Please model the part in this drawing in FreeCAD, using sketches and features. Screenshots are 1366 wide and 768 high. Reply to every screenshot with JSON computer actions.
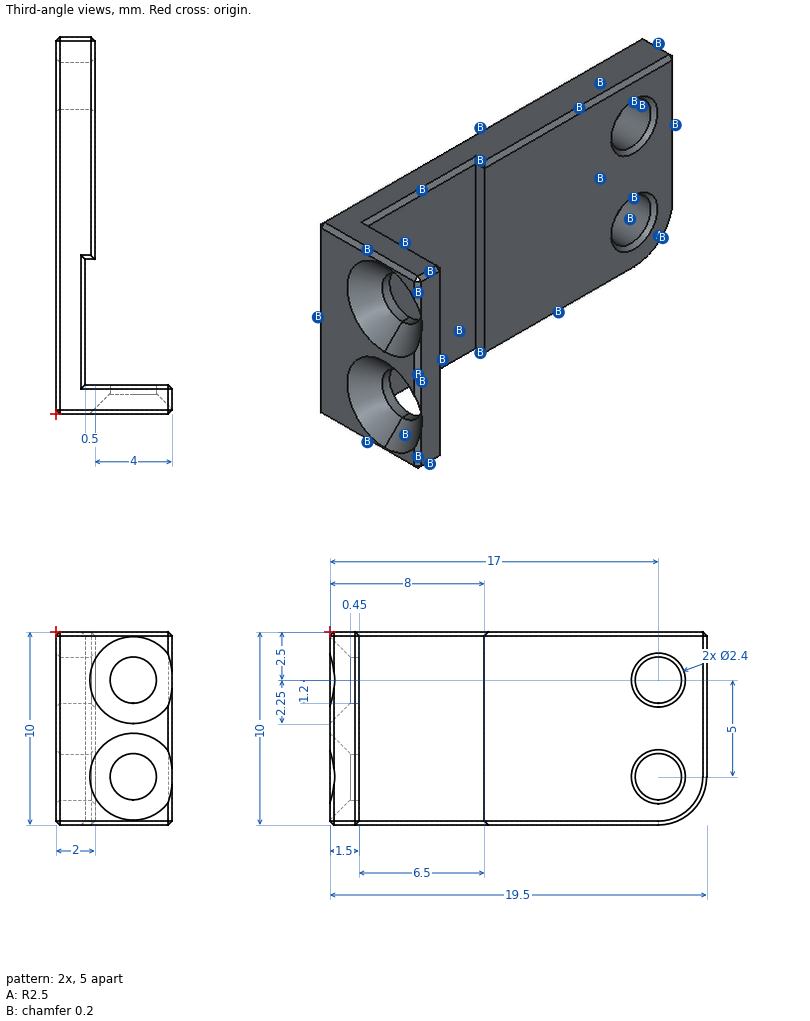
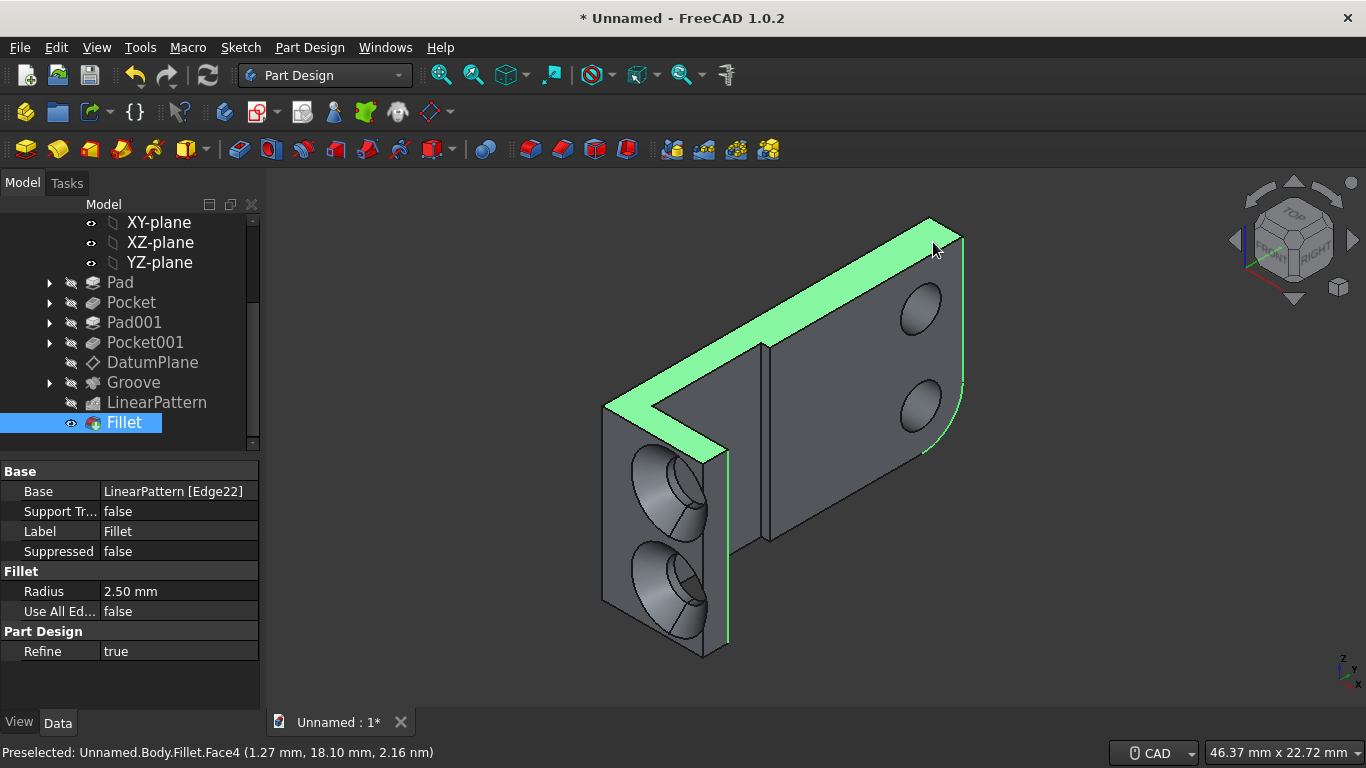
{"action": "left_click", "coordinate": [703, 560], "text": "ctrl"}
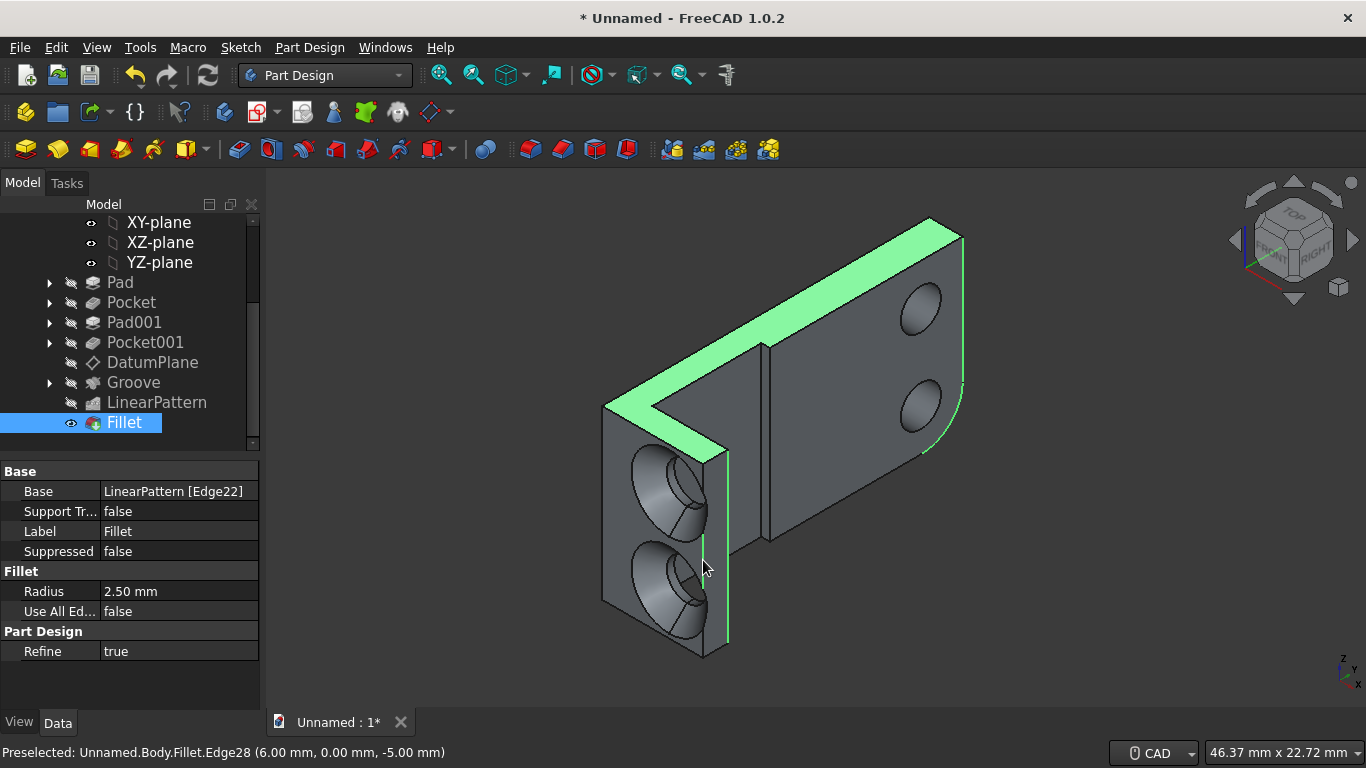
{"action": "left_click", "coordinate": [703, 643], "text": "ctrl"}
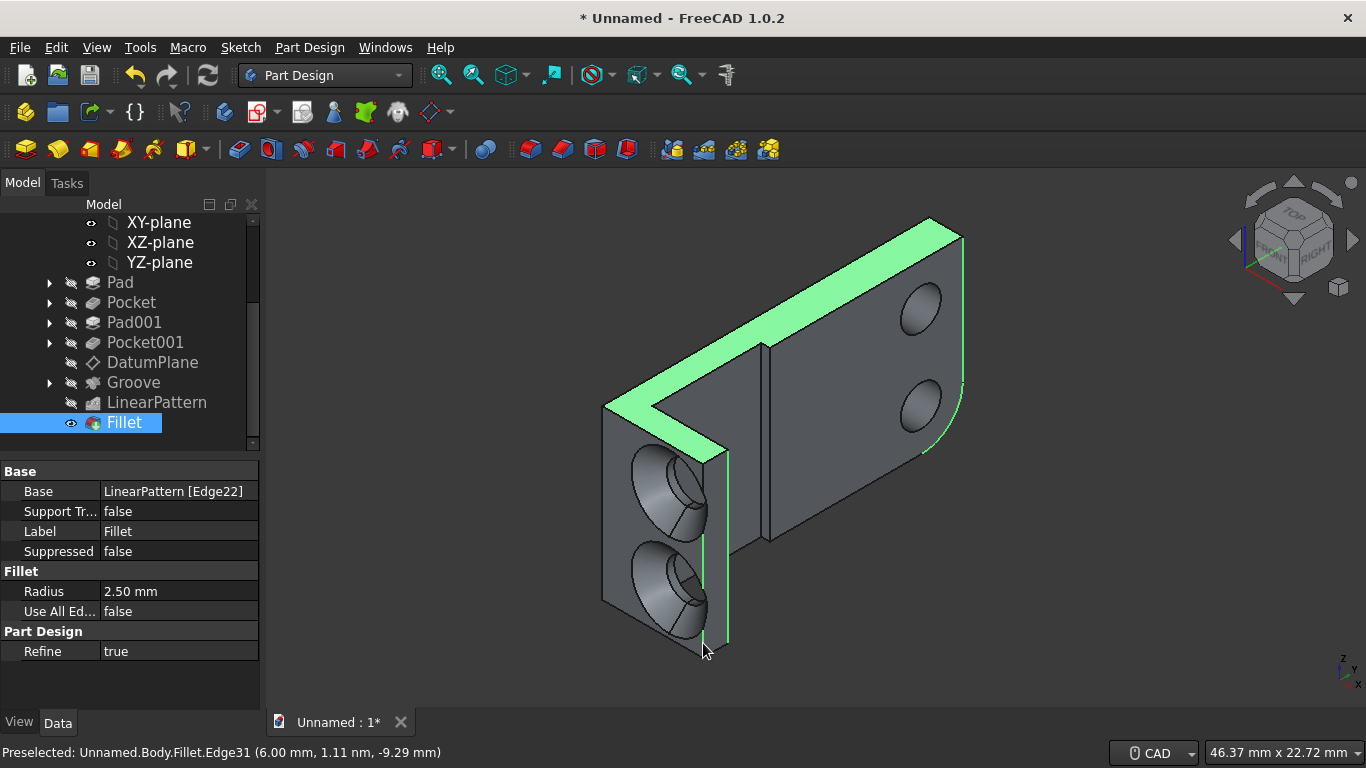
{"action": "left_click", "coordinate": [703, 477], "text": "ctrl"}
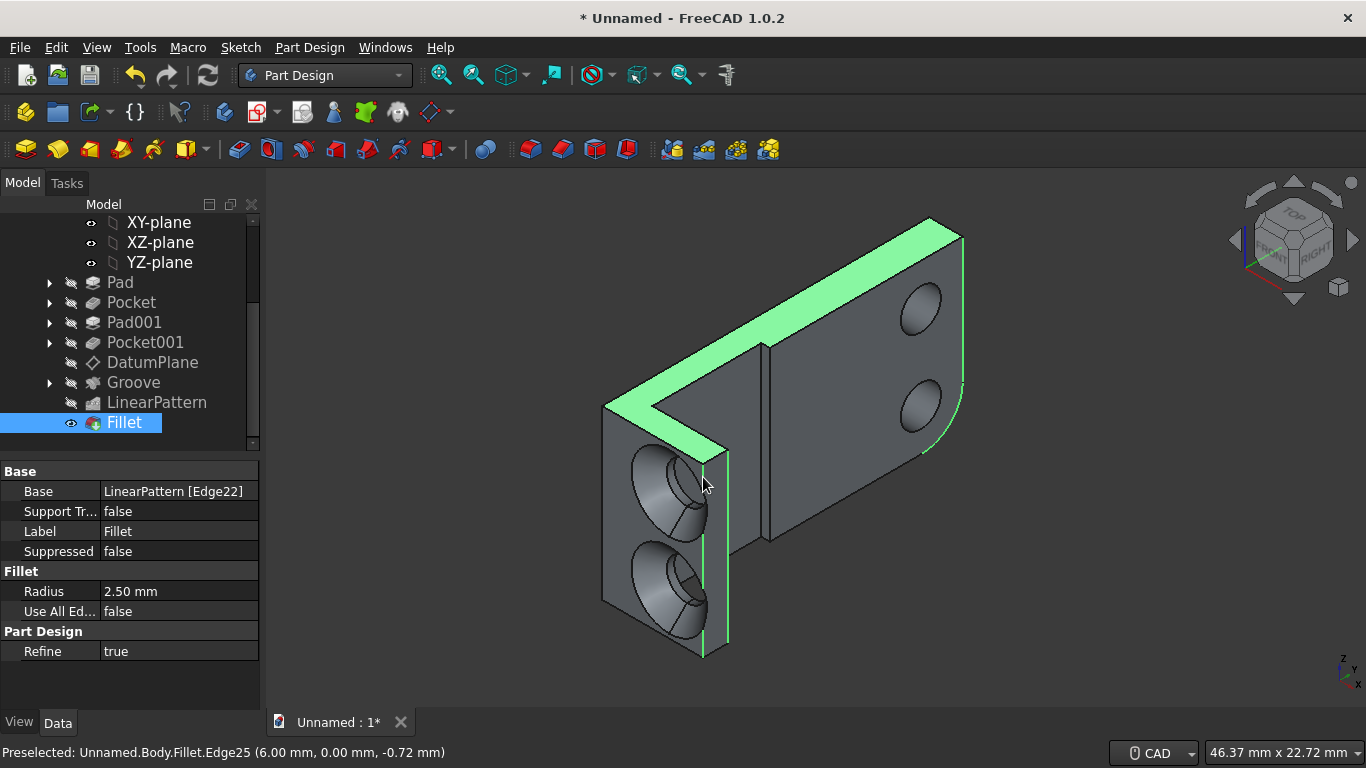
{"action": "left_click", "coordinate": [921, 331], "text": "ctrl"}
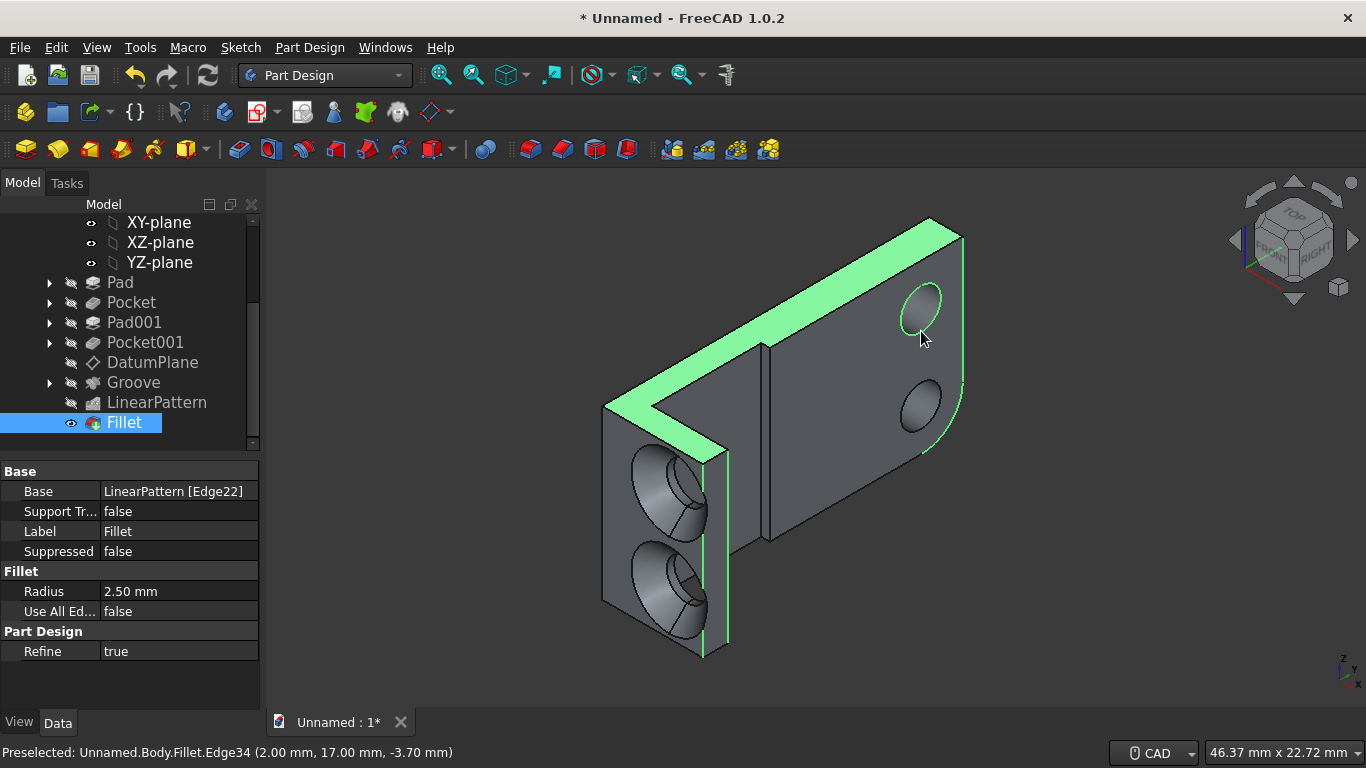
{"action": "left_click", "coordinate": [921, 428], "text": "ctrl"}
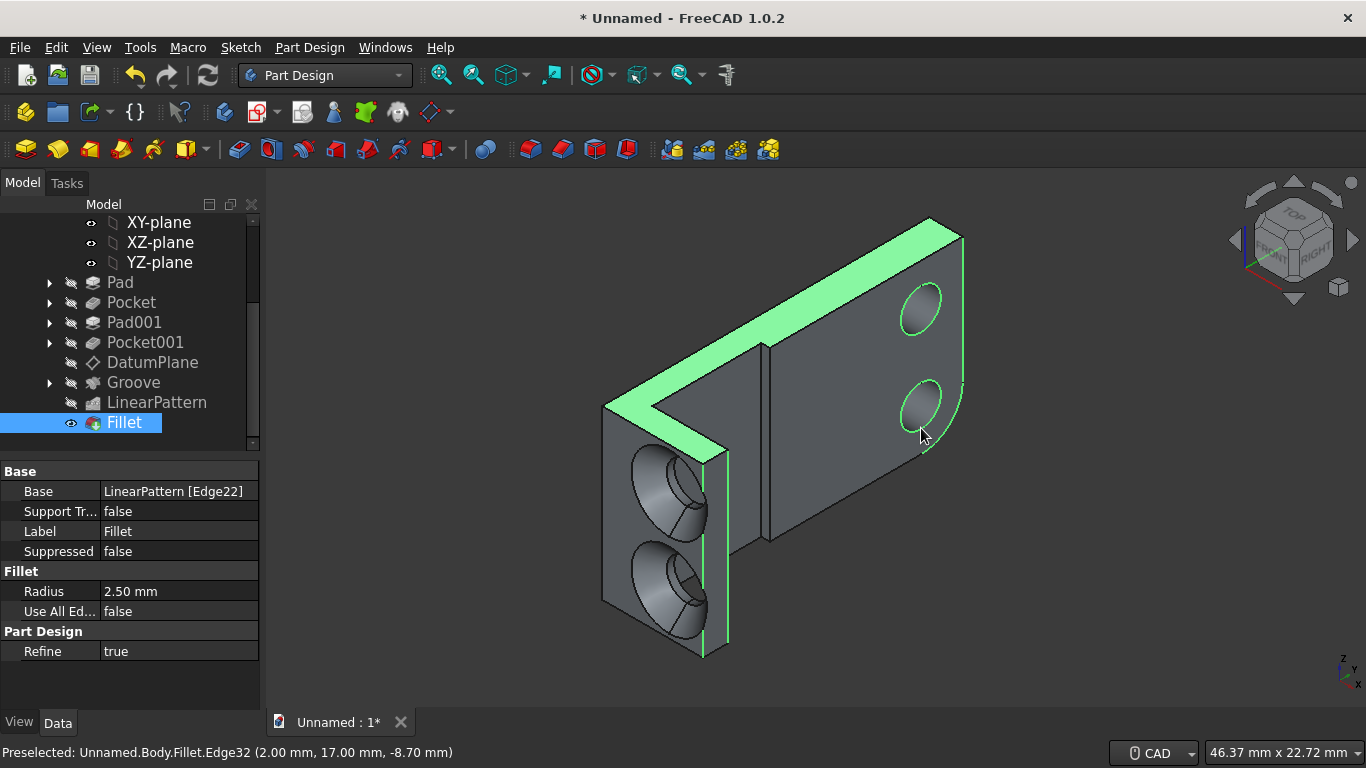
{"action": "key", "text": "2"}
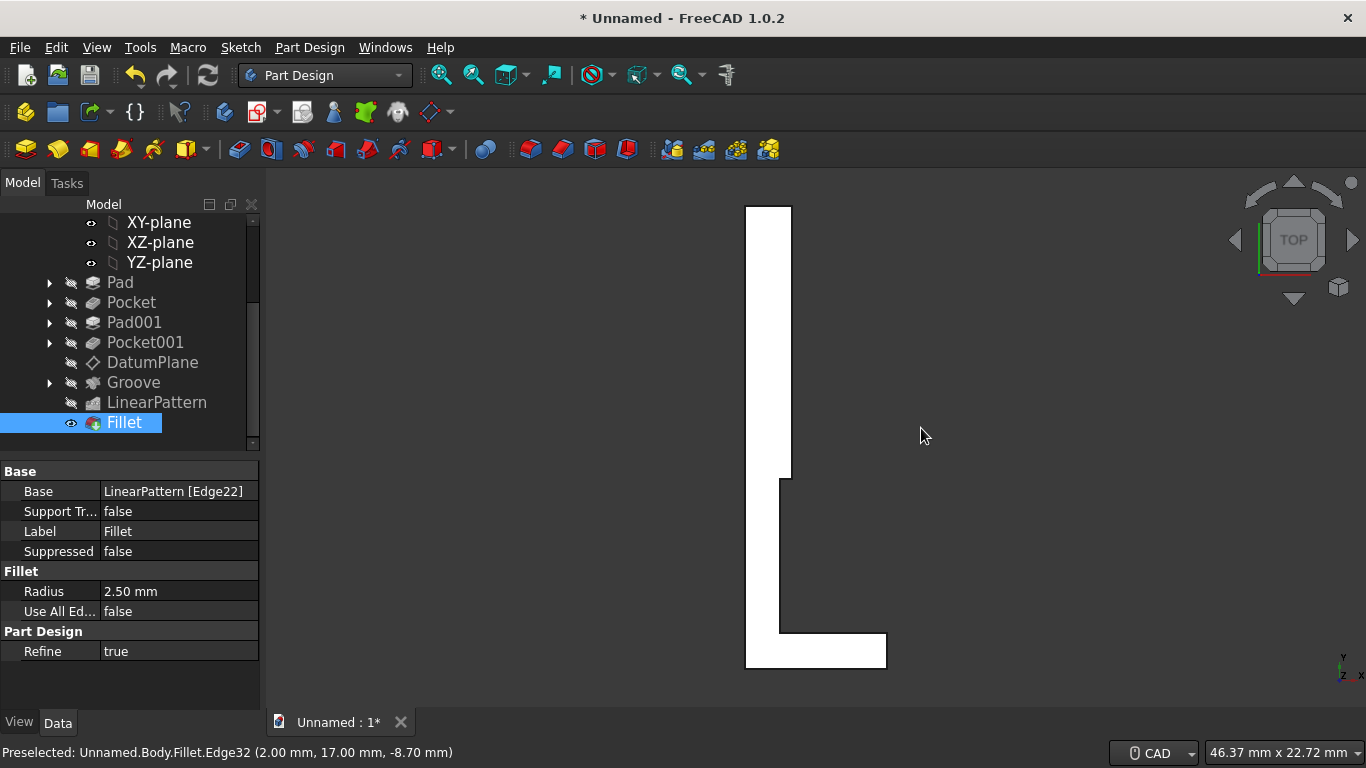
{"action": "key", "text": "1"}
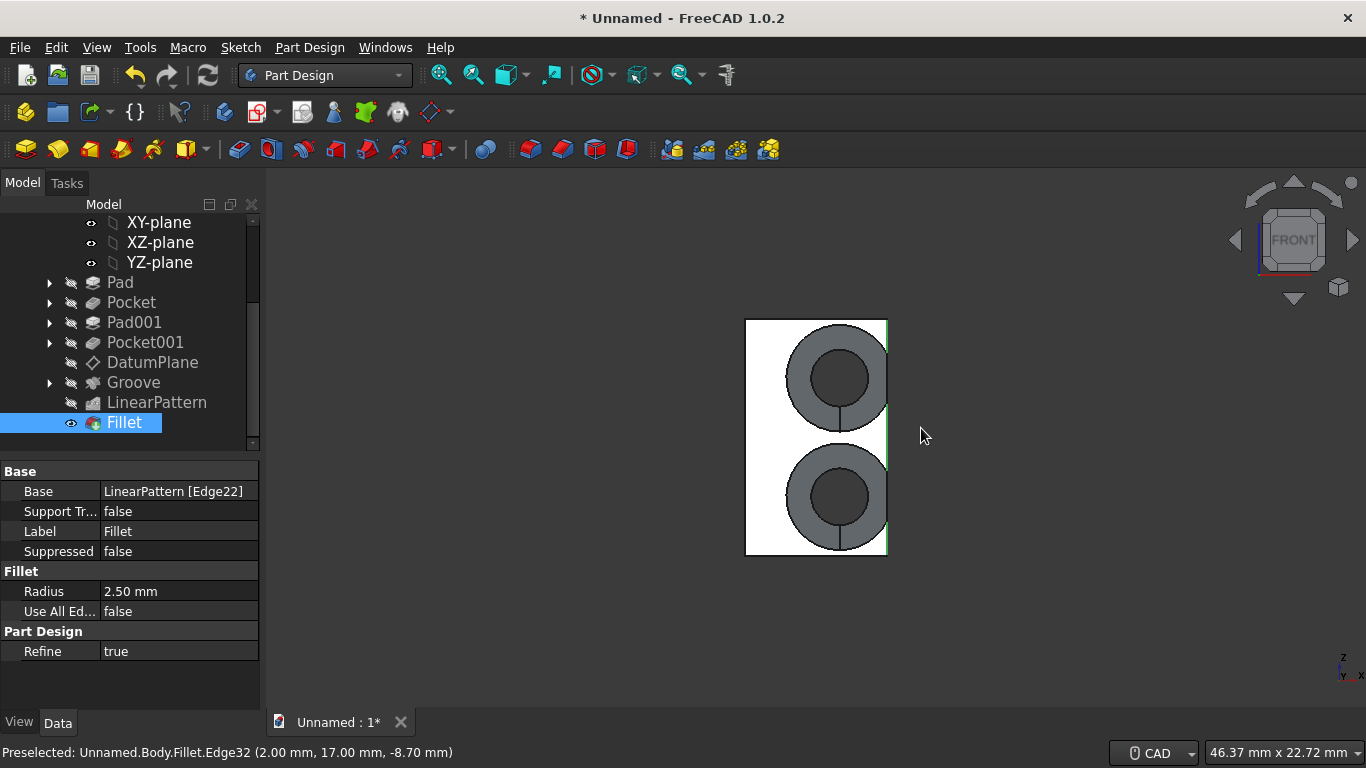
{"action": "left_click", "coordinate": [442, 76]}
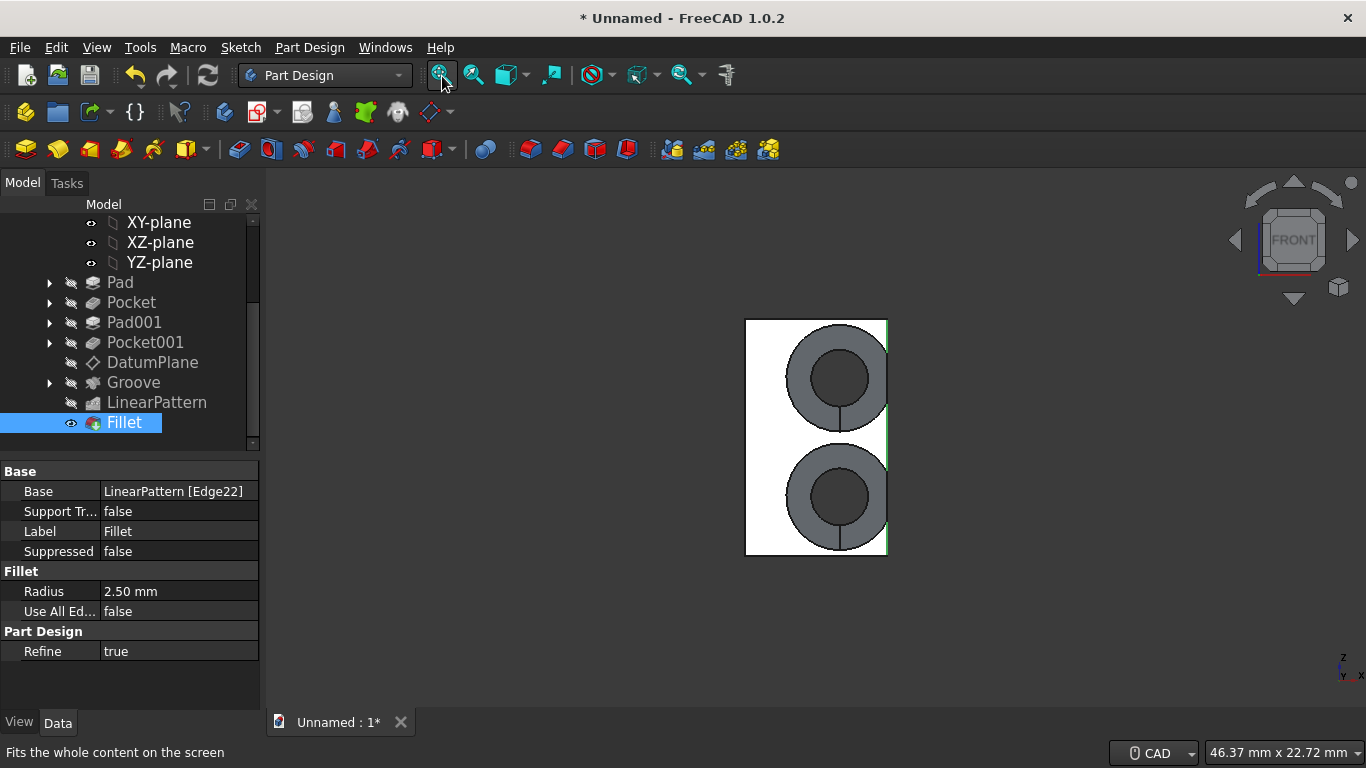
{"action": "key", "text": "3"}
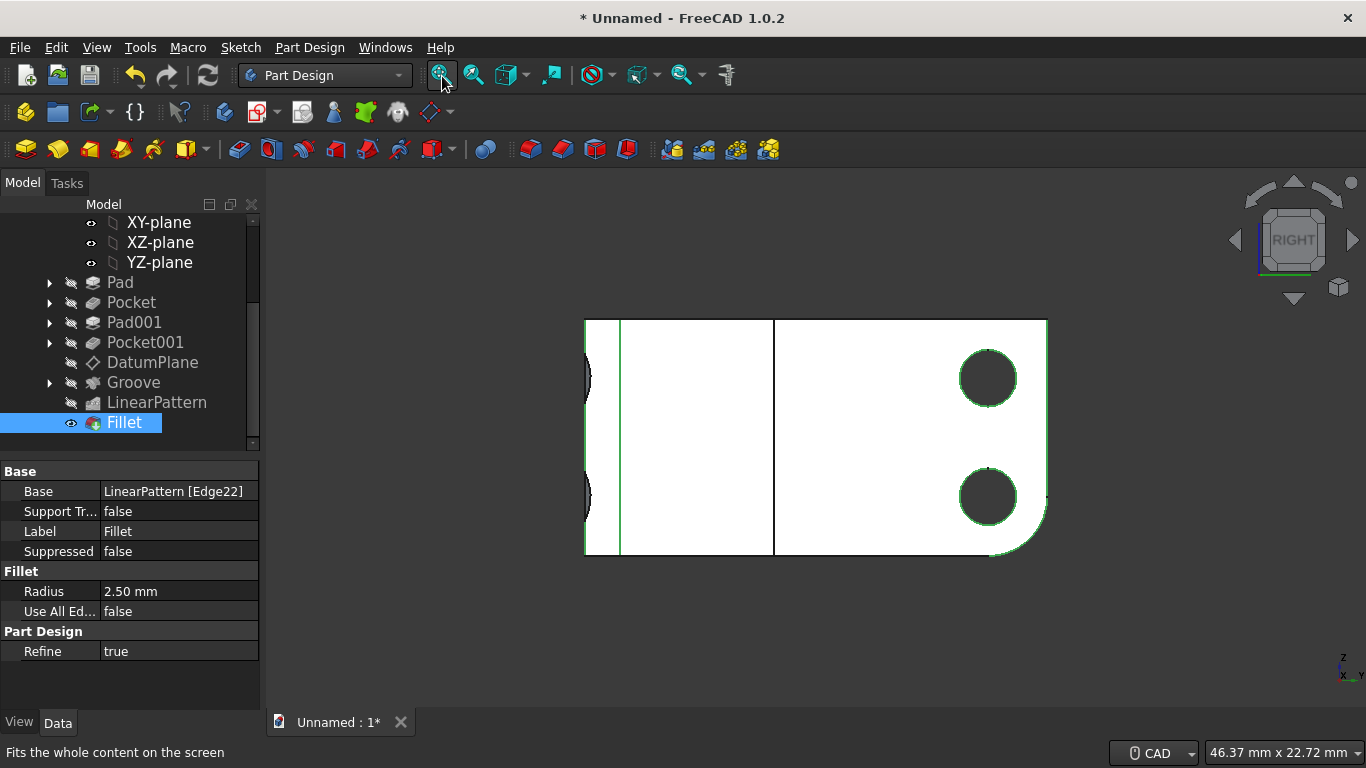
{"action": "left_click", "coordinate": [442, 76]}